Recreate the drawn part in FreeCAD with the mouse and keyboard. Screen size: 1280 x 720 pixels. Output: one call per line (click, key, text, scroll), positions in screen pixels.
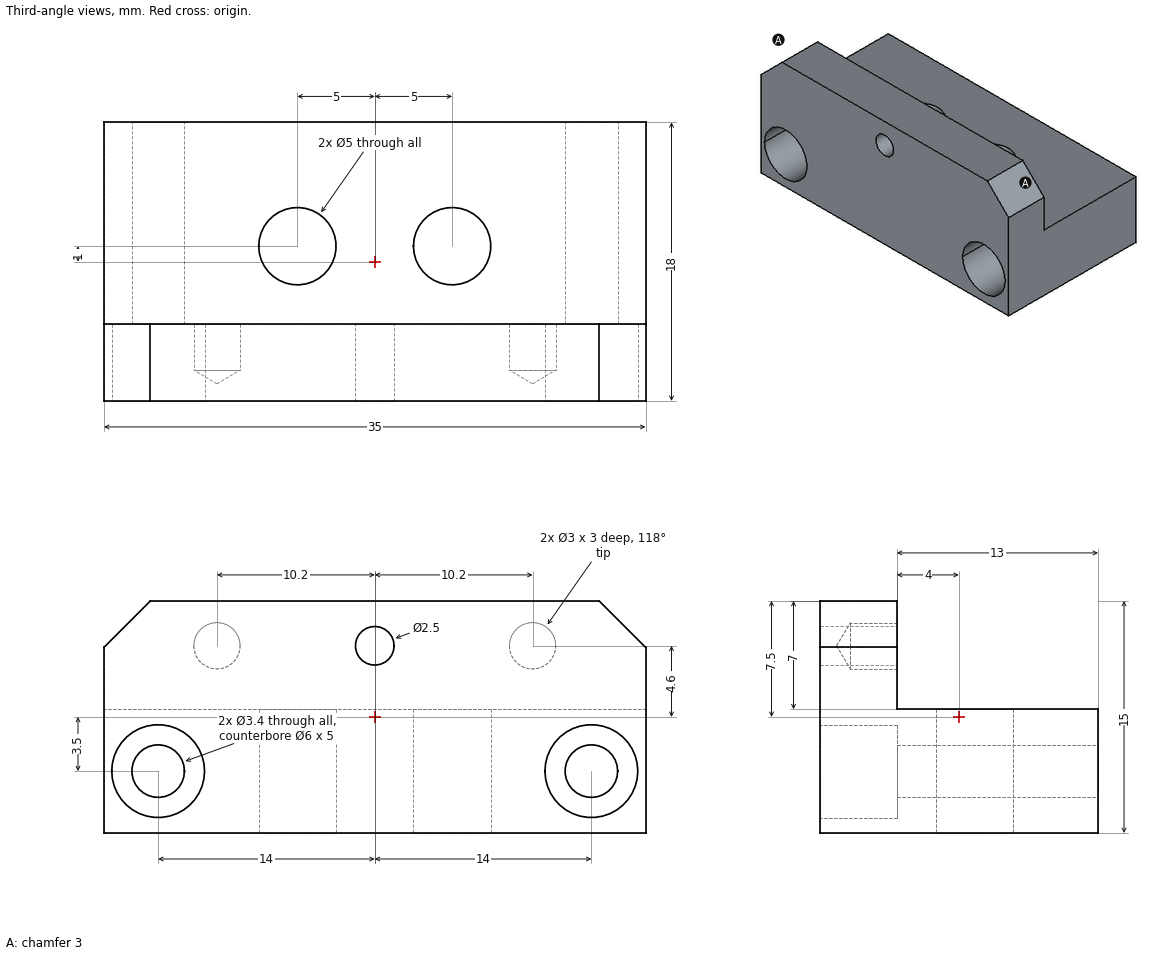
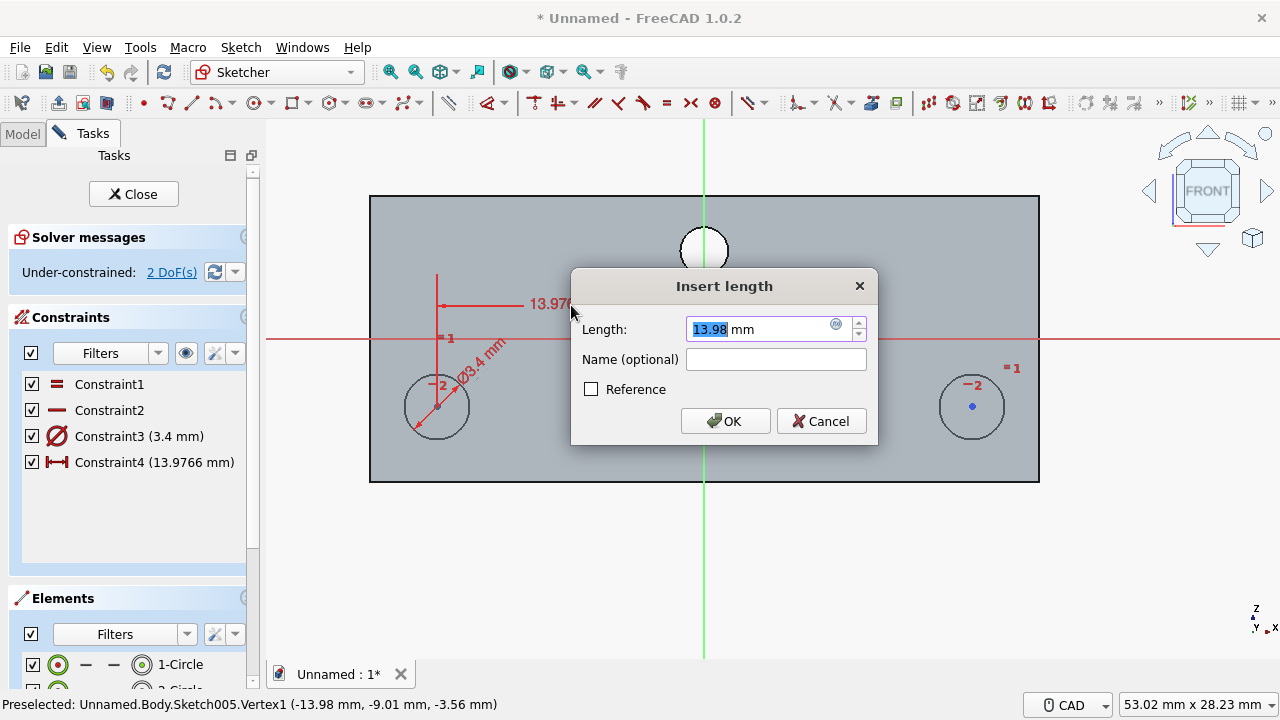
text(14)
key(Return)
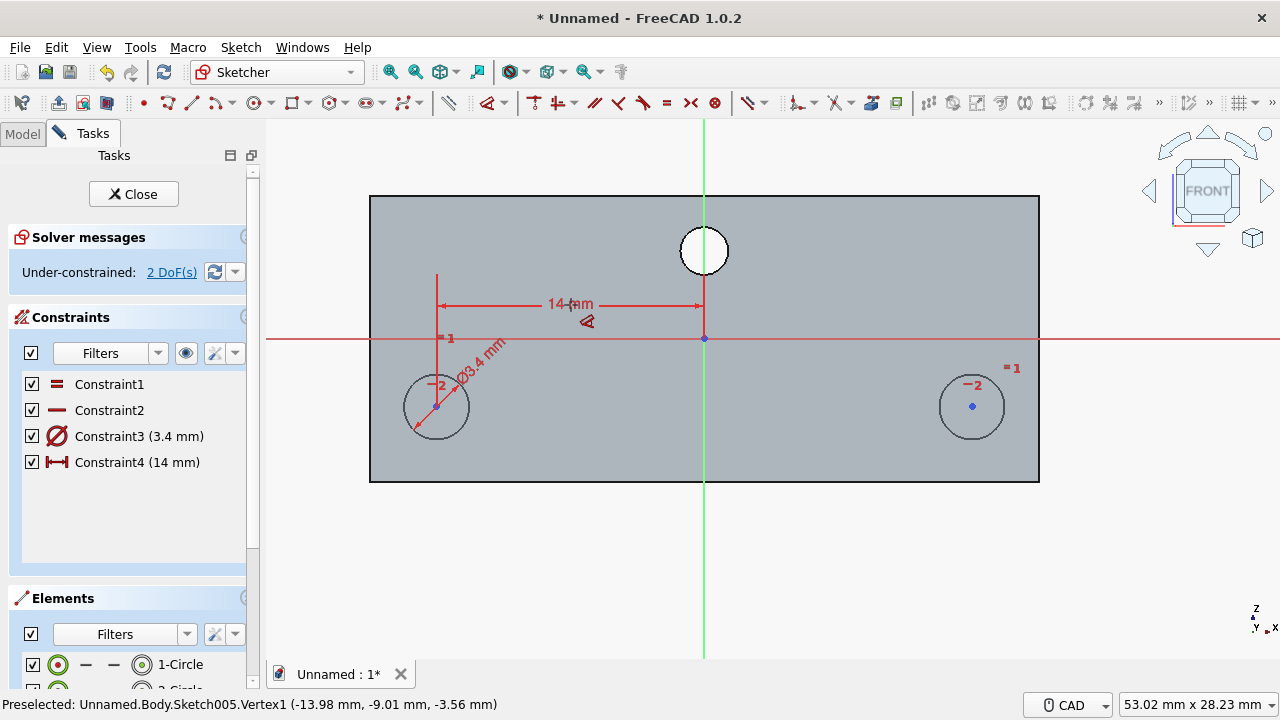
click(972, 407)
click(838, 305)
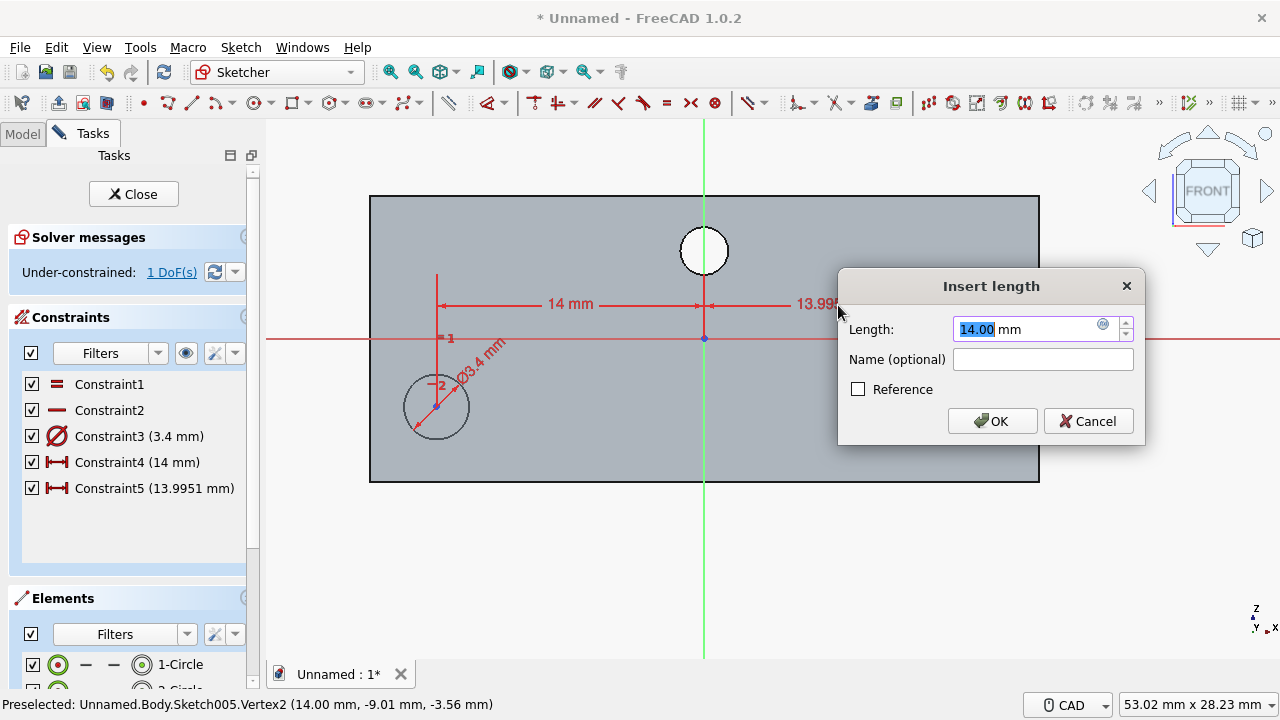
text(14)
key(Return)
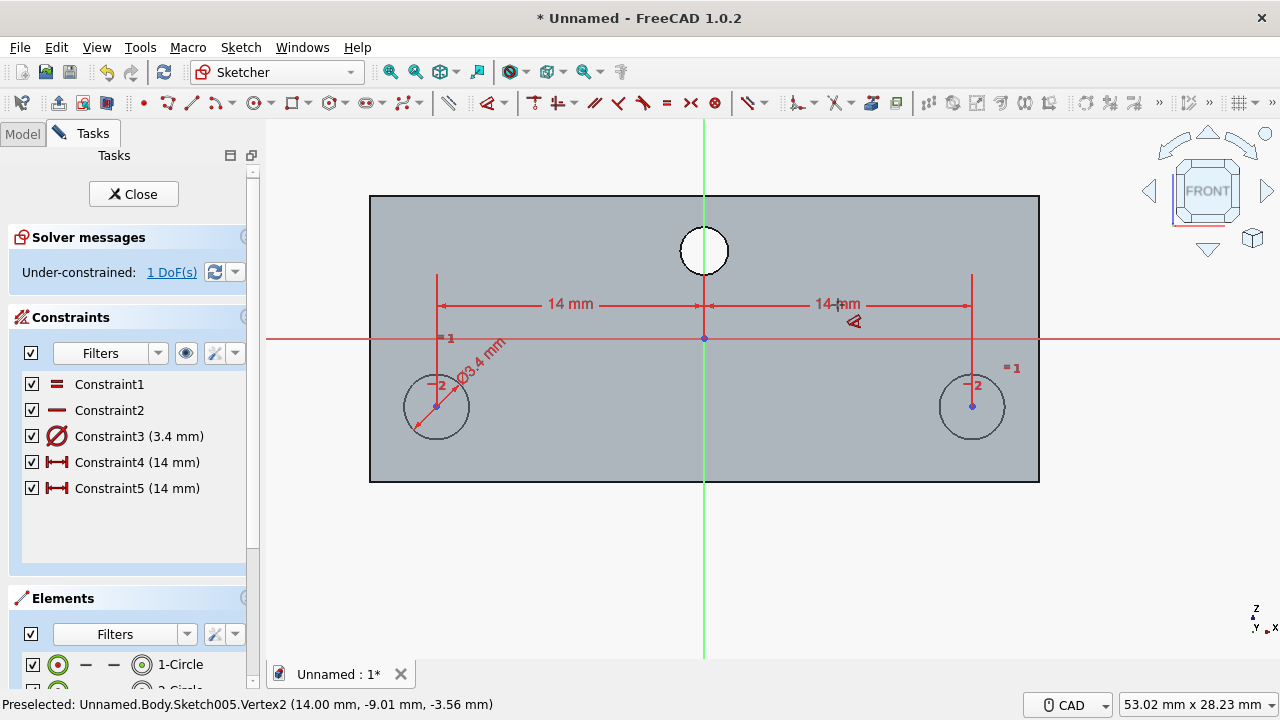
click(437, 407)
click(403, 373)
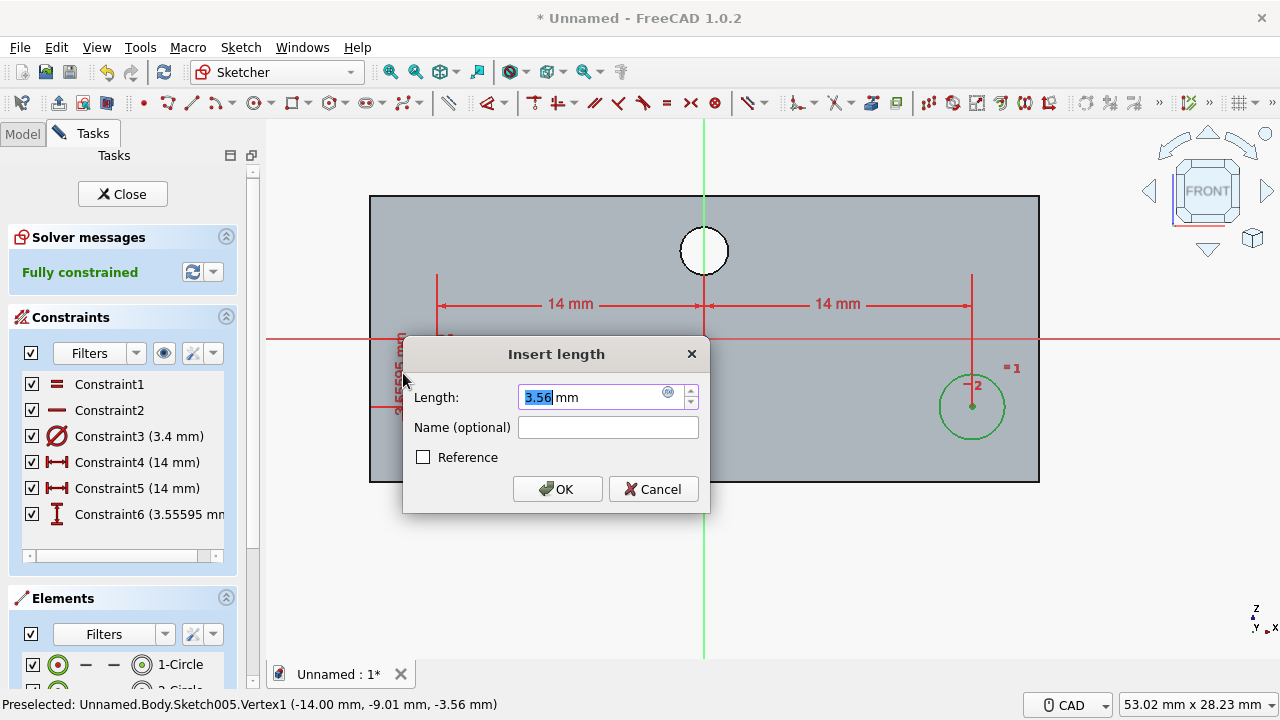
text(3.5)
key(Return)
key(Escape)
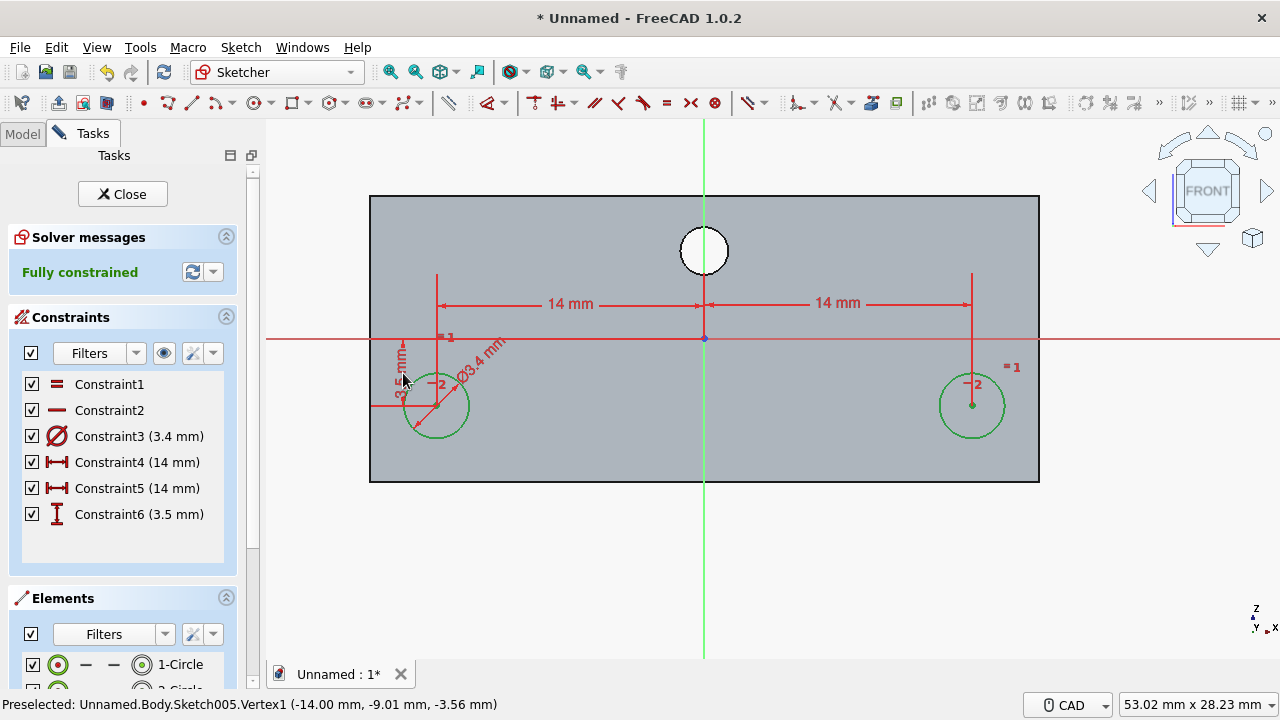
click(123, 194)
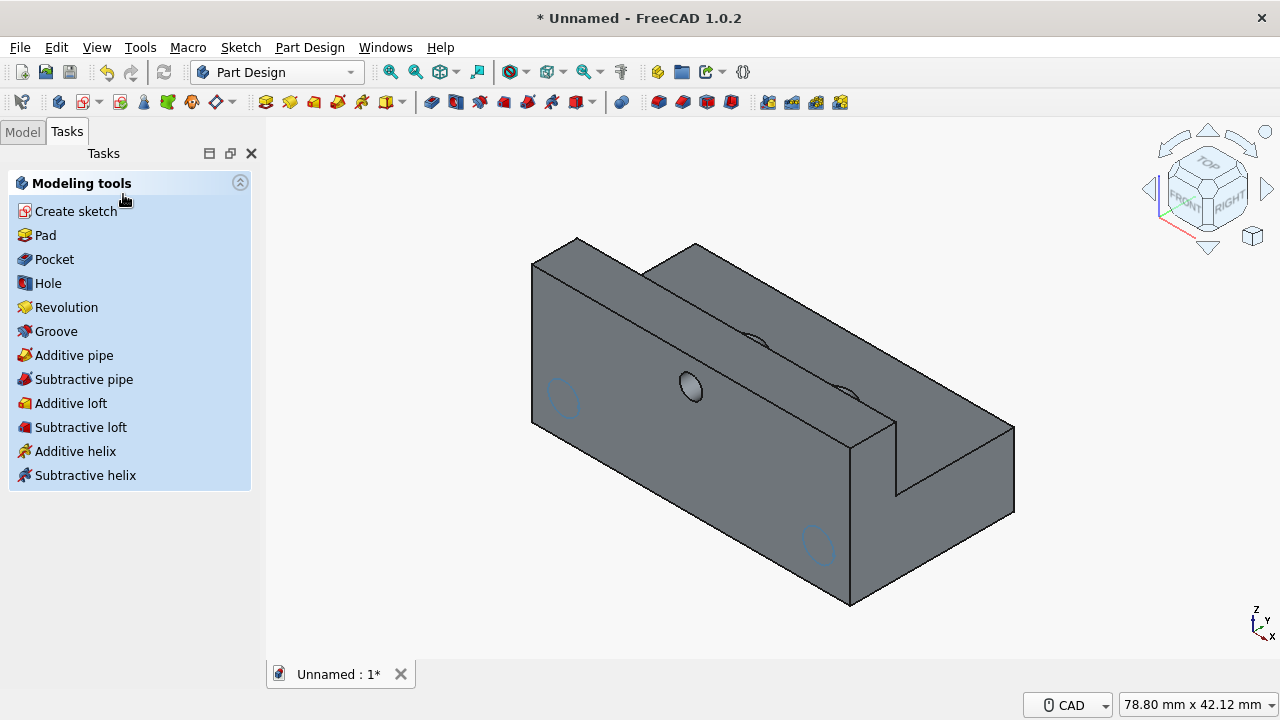
click(456, 102)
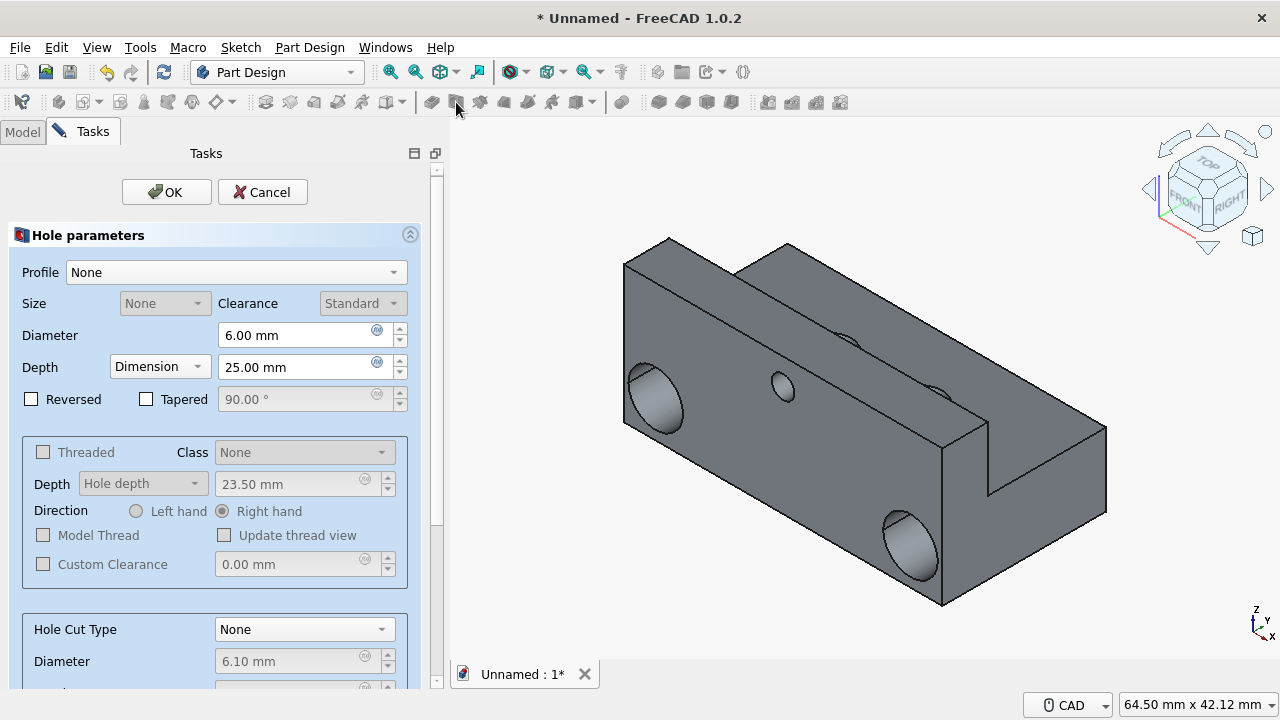
triple_click(305, 335)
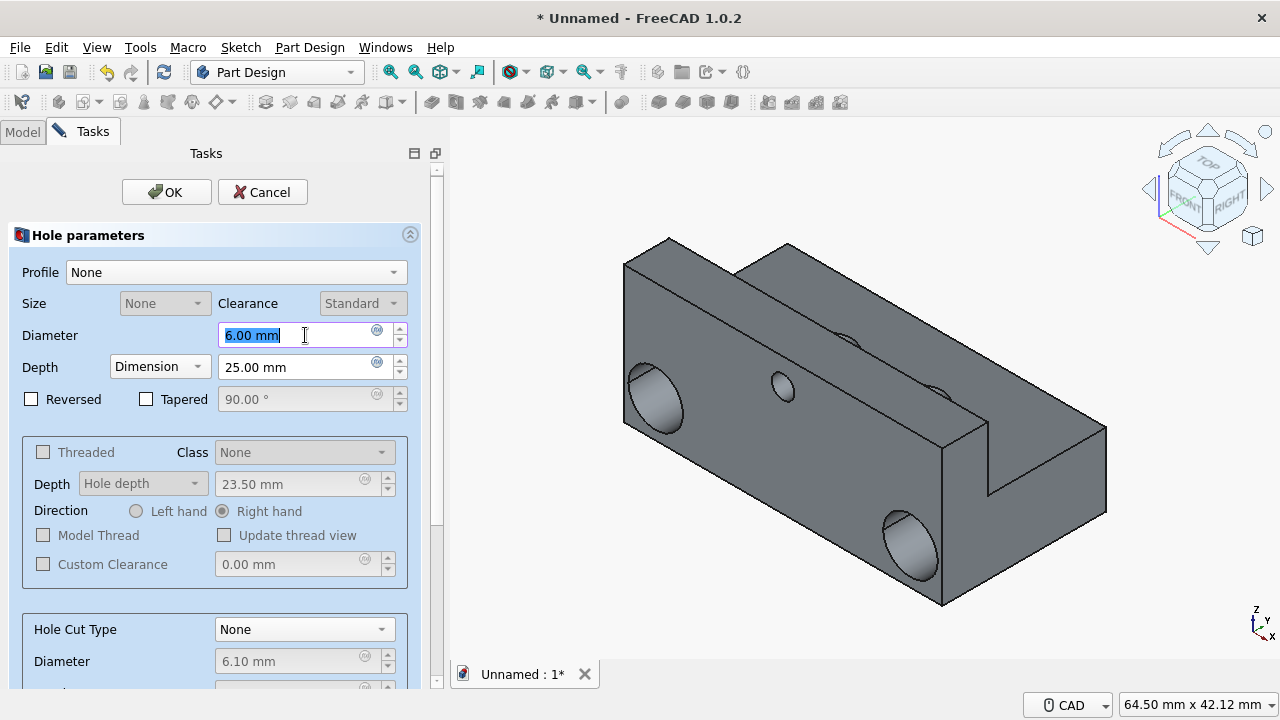
text(3.4)
key(Tab)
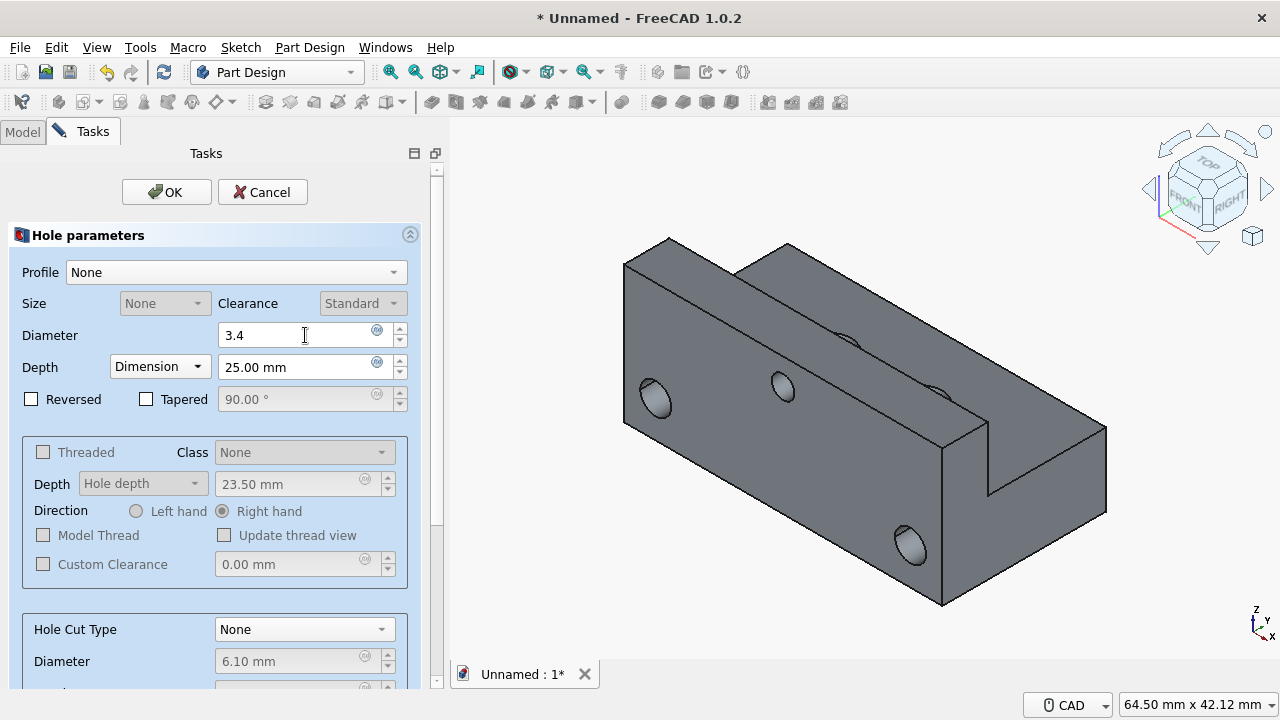
click(161, 366)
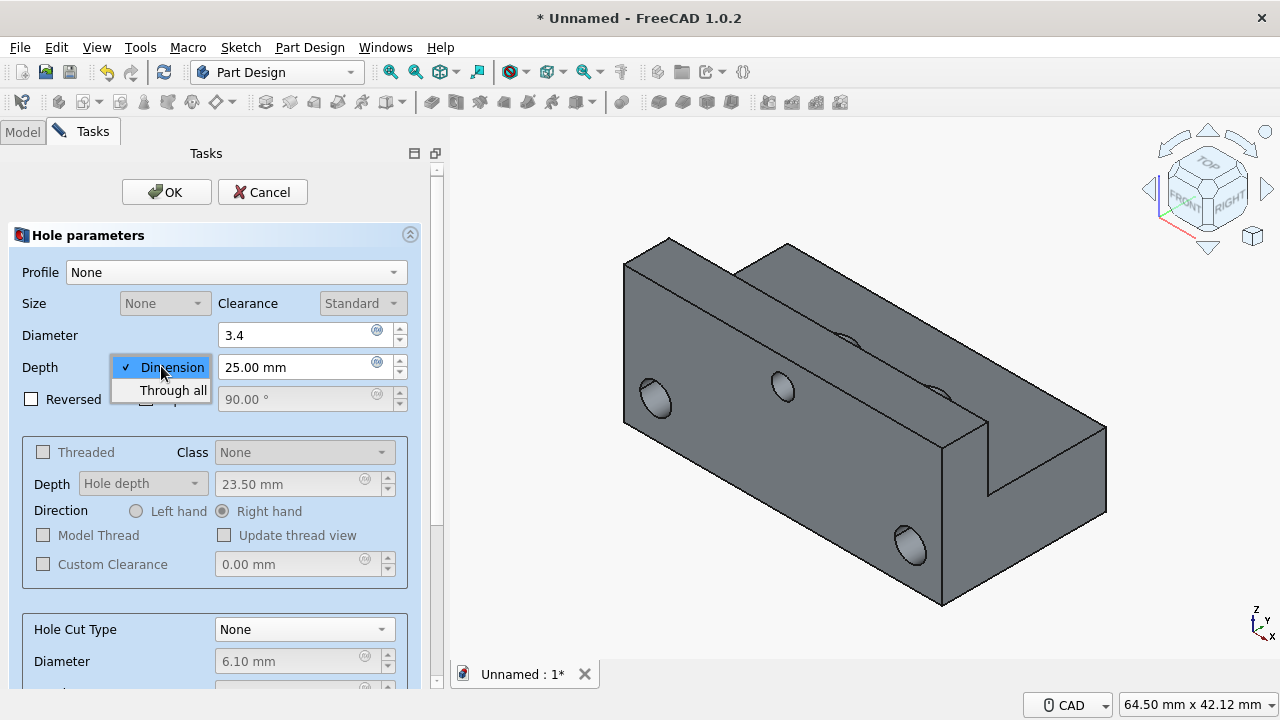
click(160, 390)